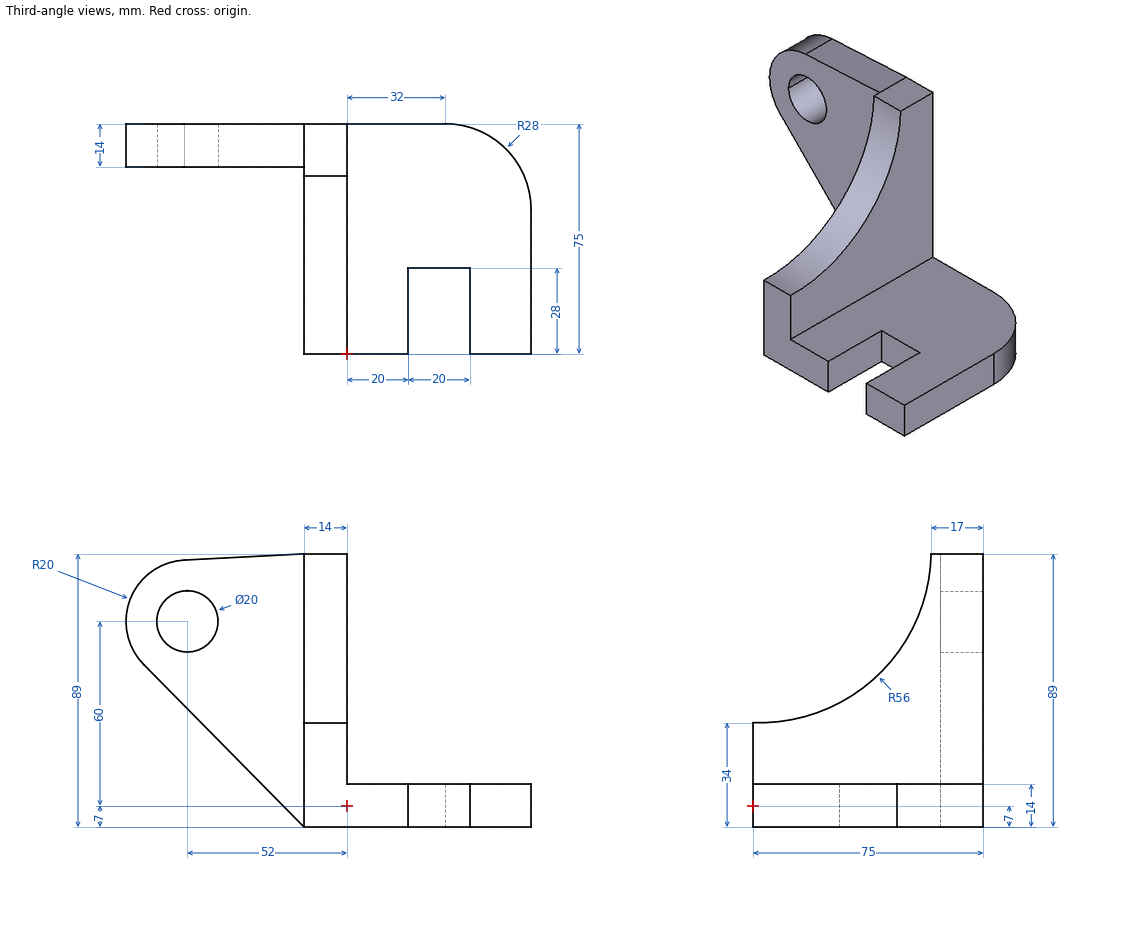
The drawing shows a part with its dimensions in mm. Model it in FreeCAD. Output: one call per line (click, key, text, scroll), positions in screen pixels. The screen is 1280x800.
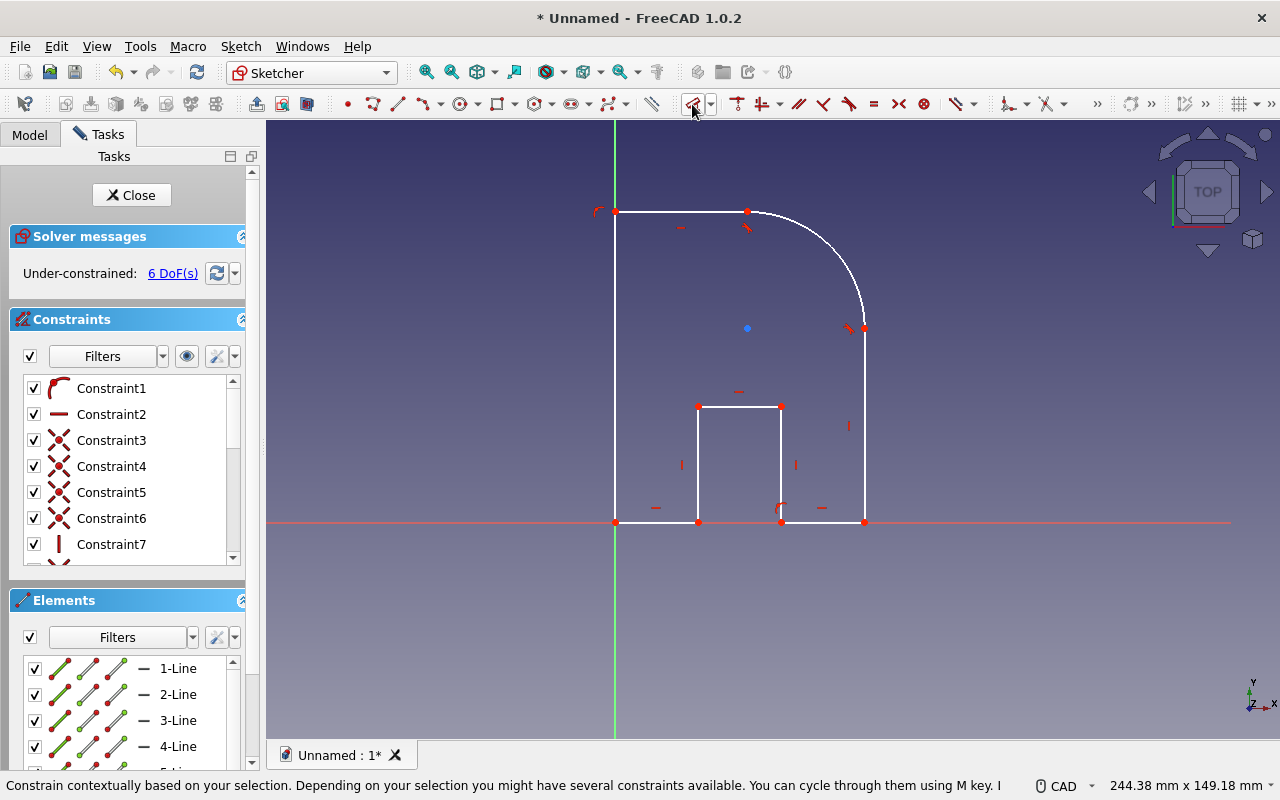
click(852, 276)
click(881, 262)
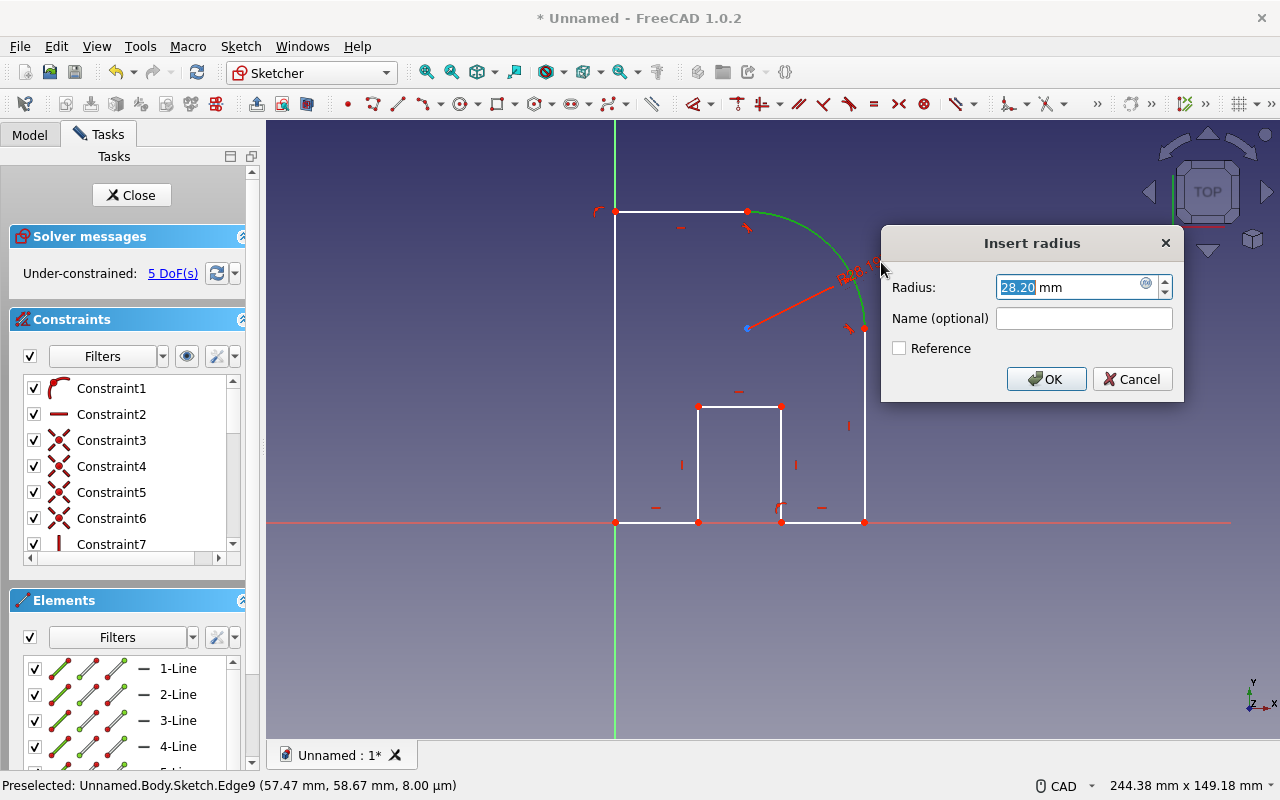
text(28)
key(Return)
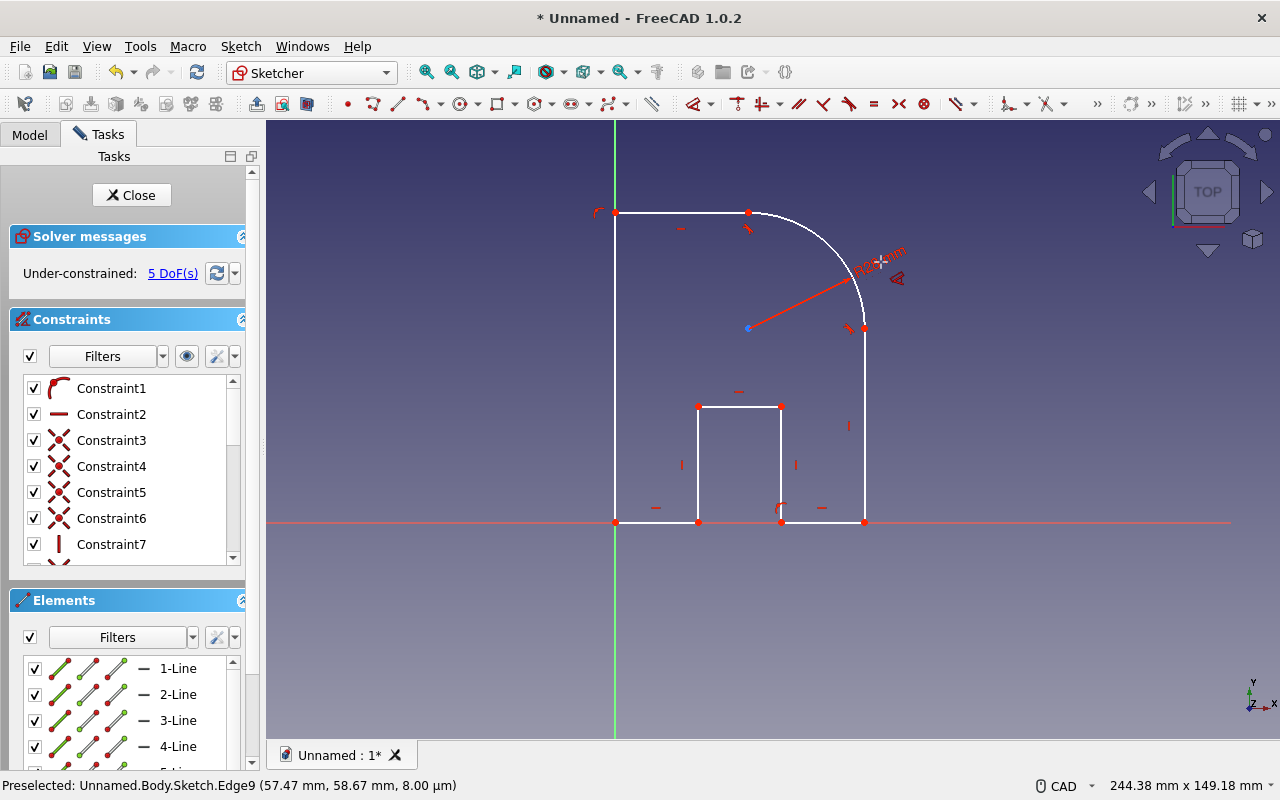
click(708, 213)
click(682, 179)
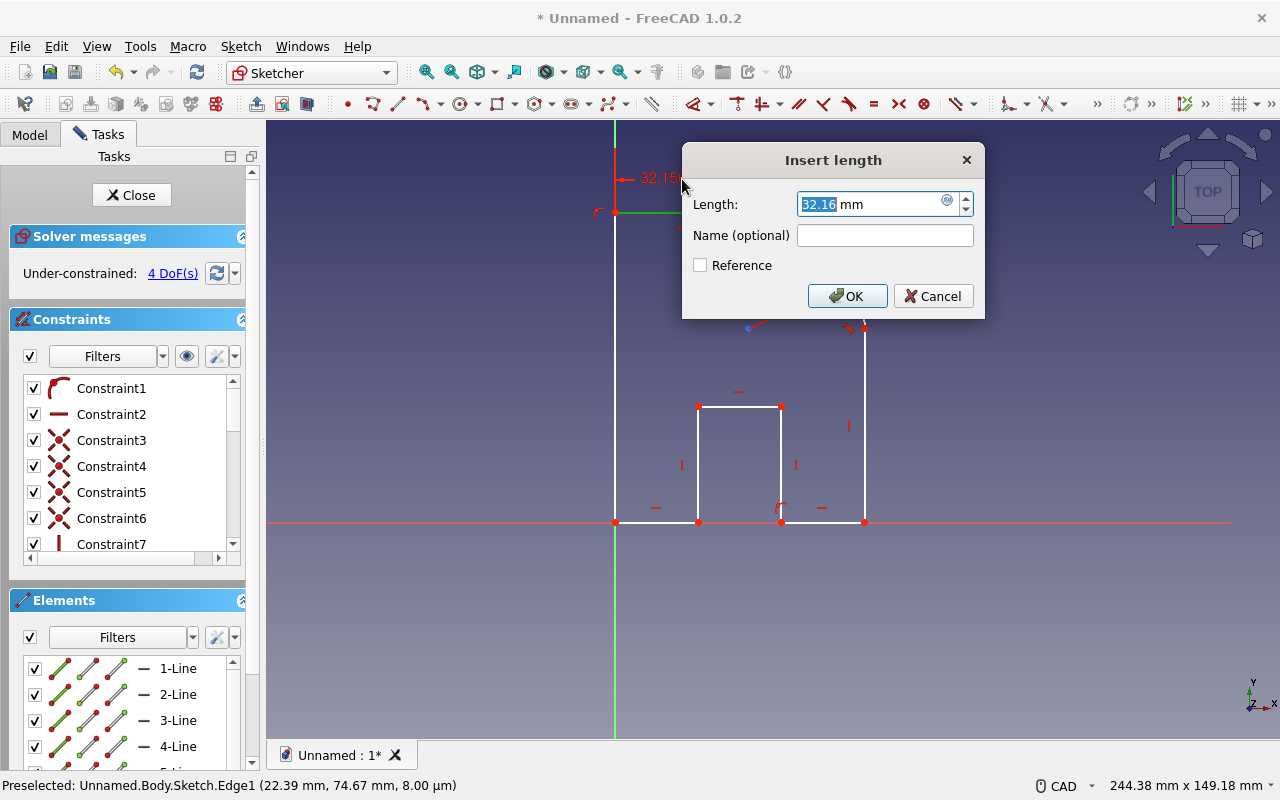
text(32)
key(Return)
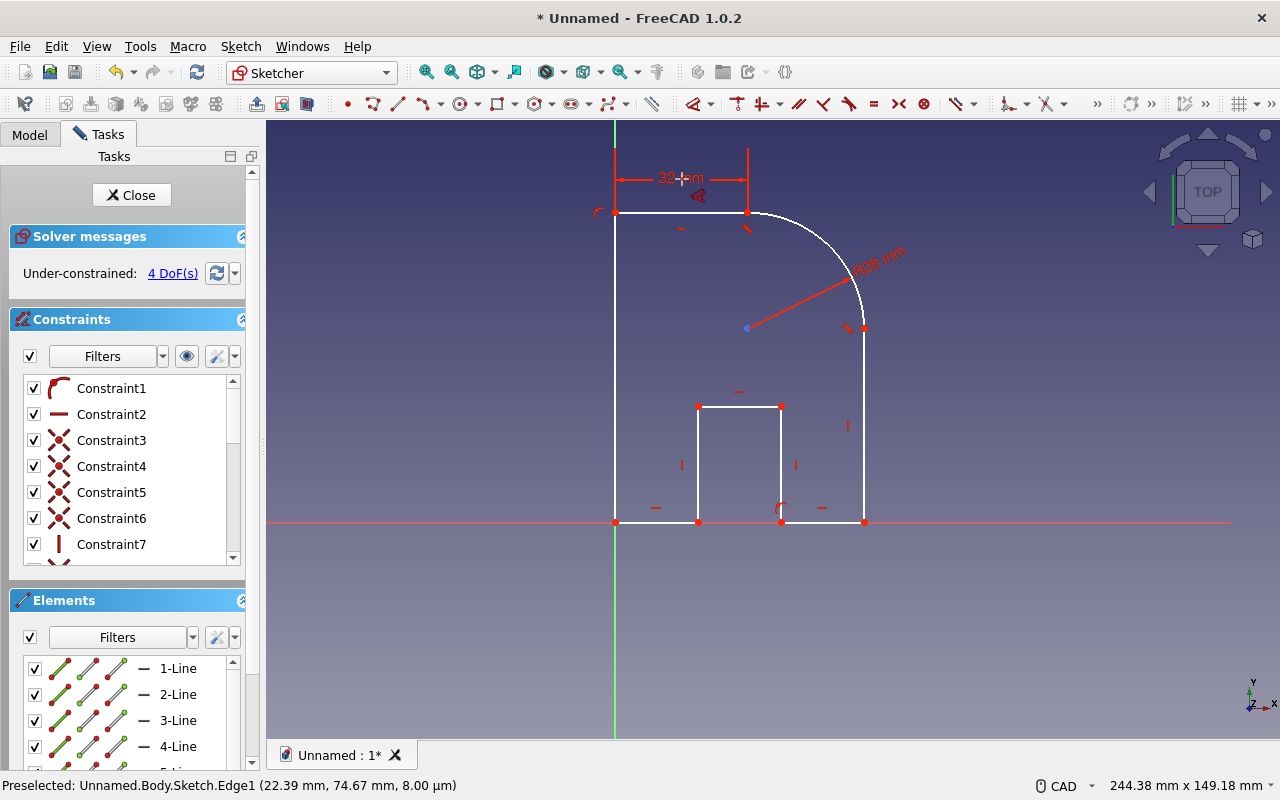
click(615, 306)
click(581, 368)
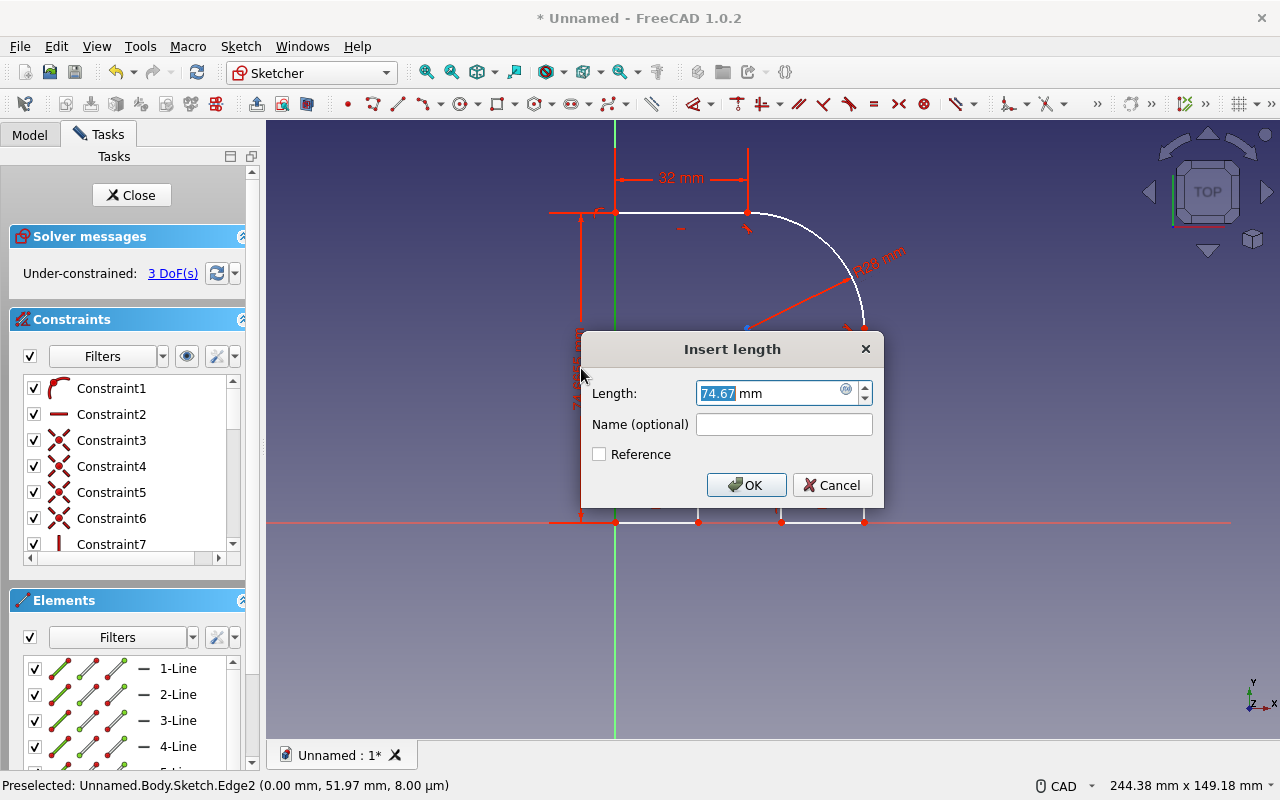
text(75)
key(Return)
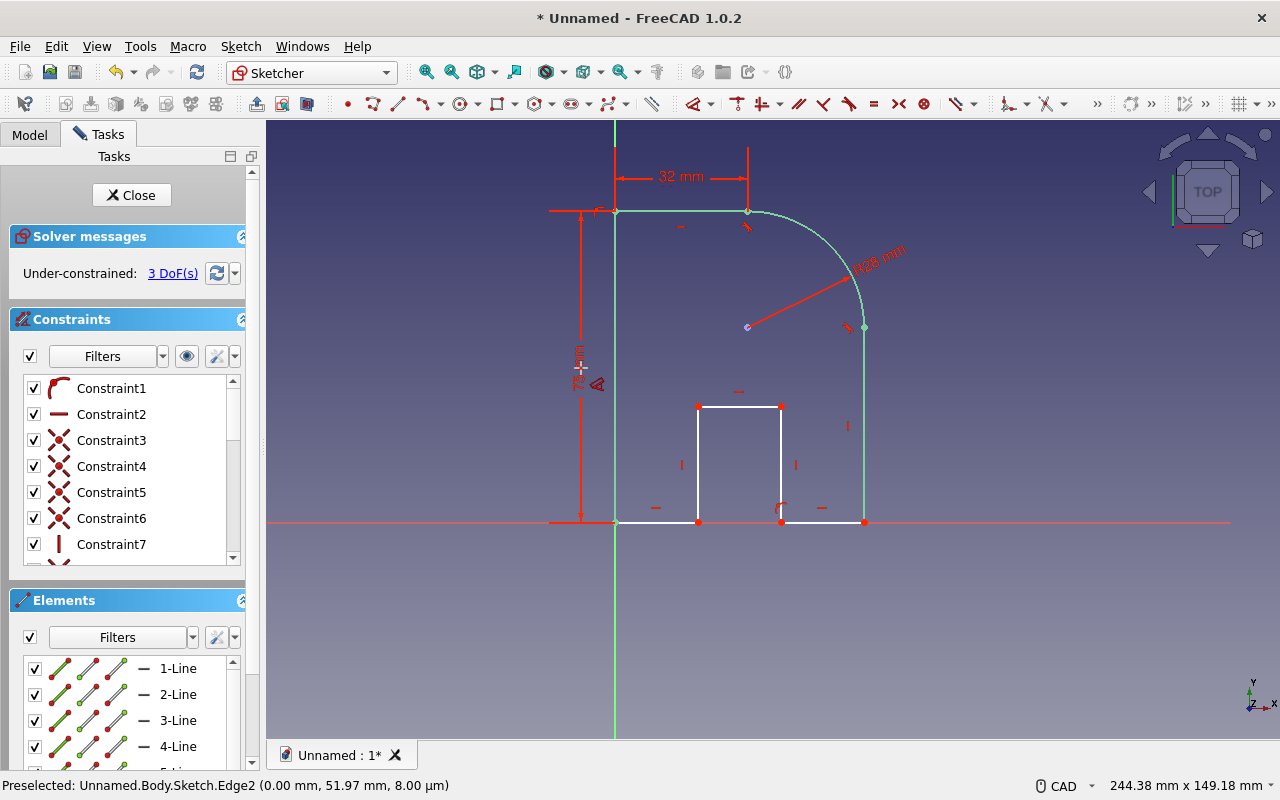
click(640, 523)
click(657, 557)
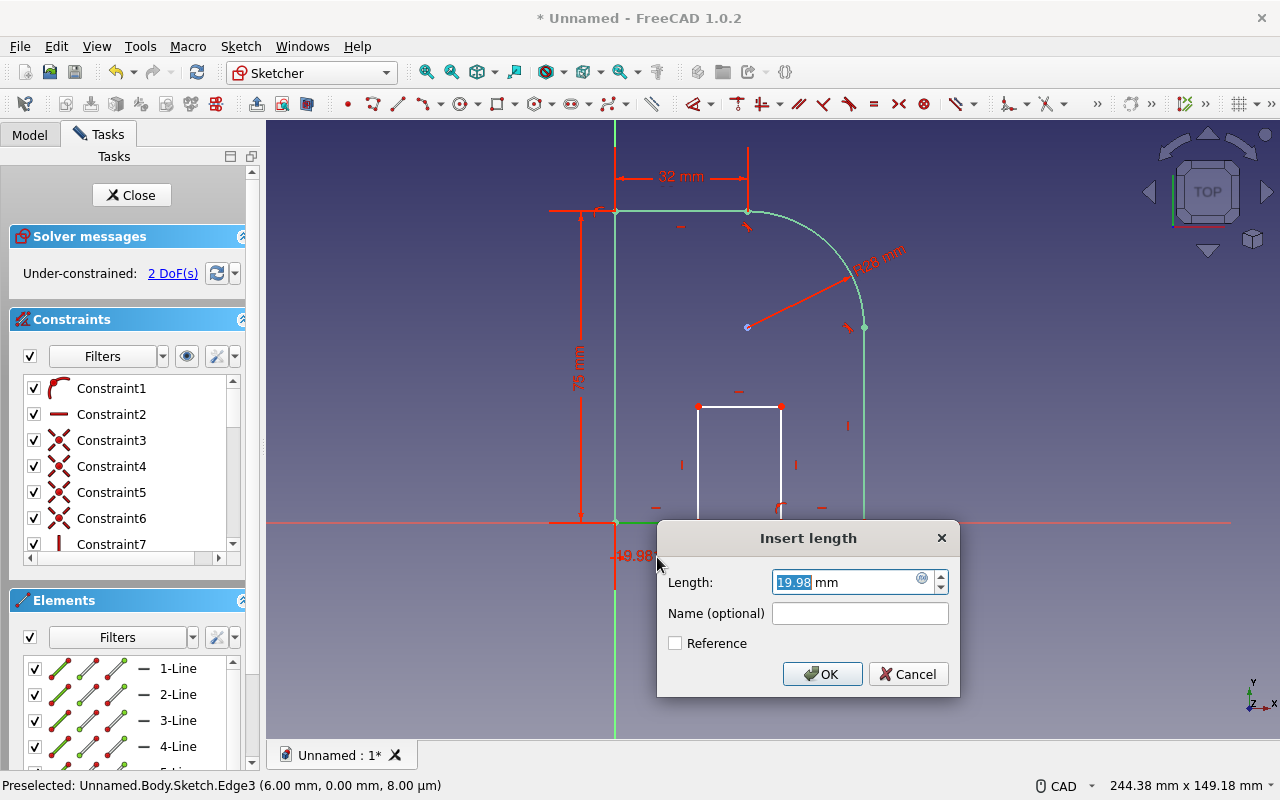
text(20)
key(Return)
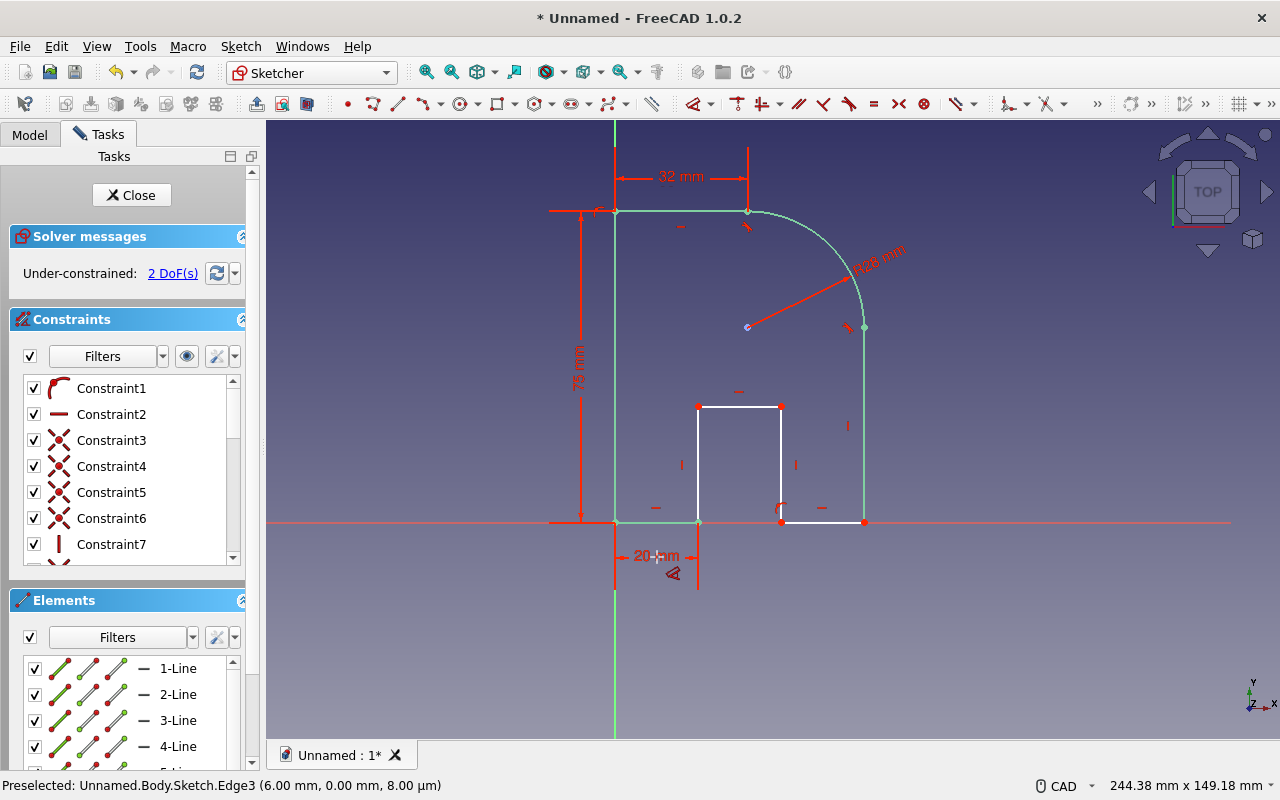
click(698, 488)
click(664, 465)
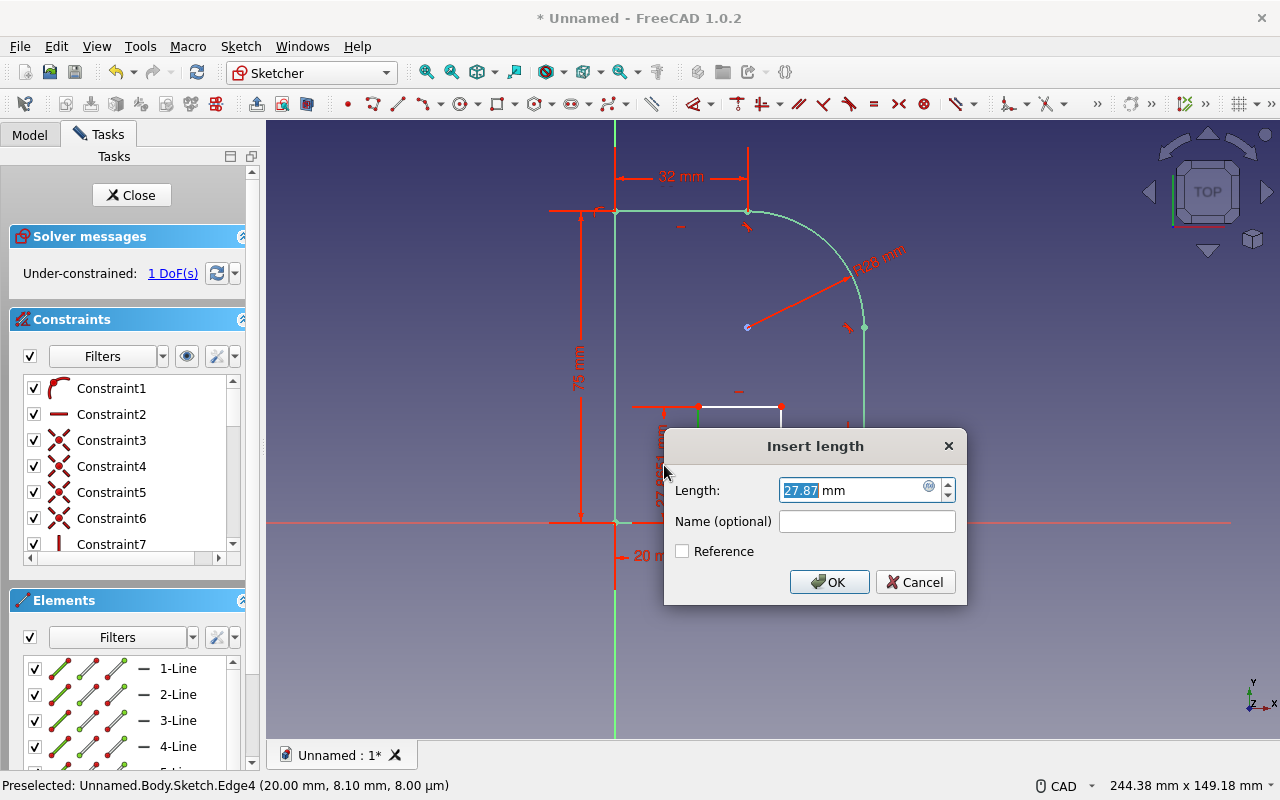
text(28)
key(Return)